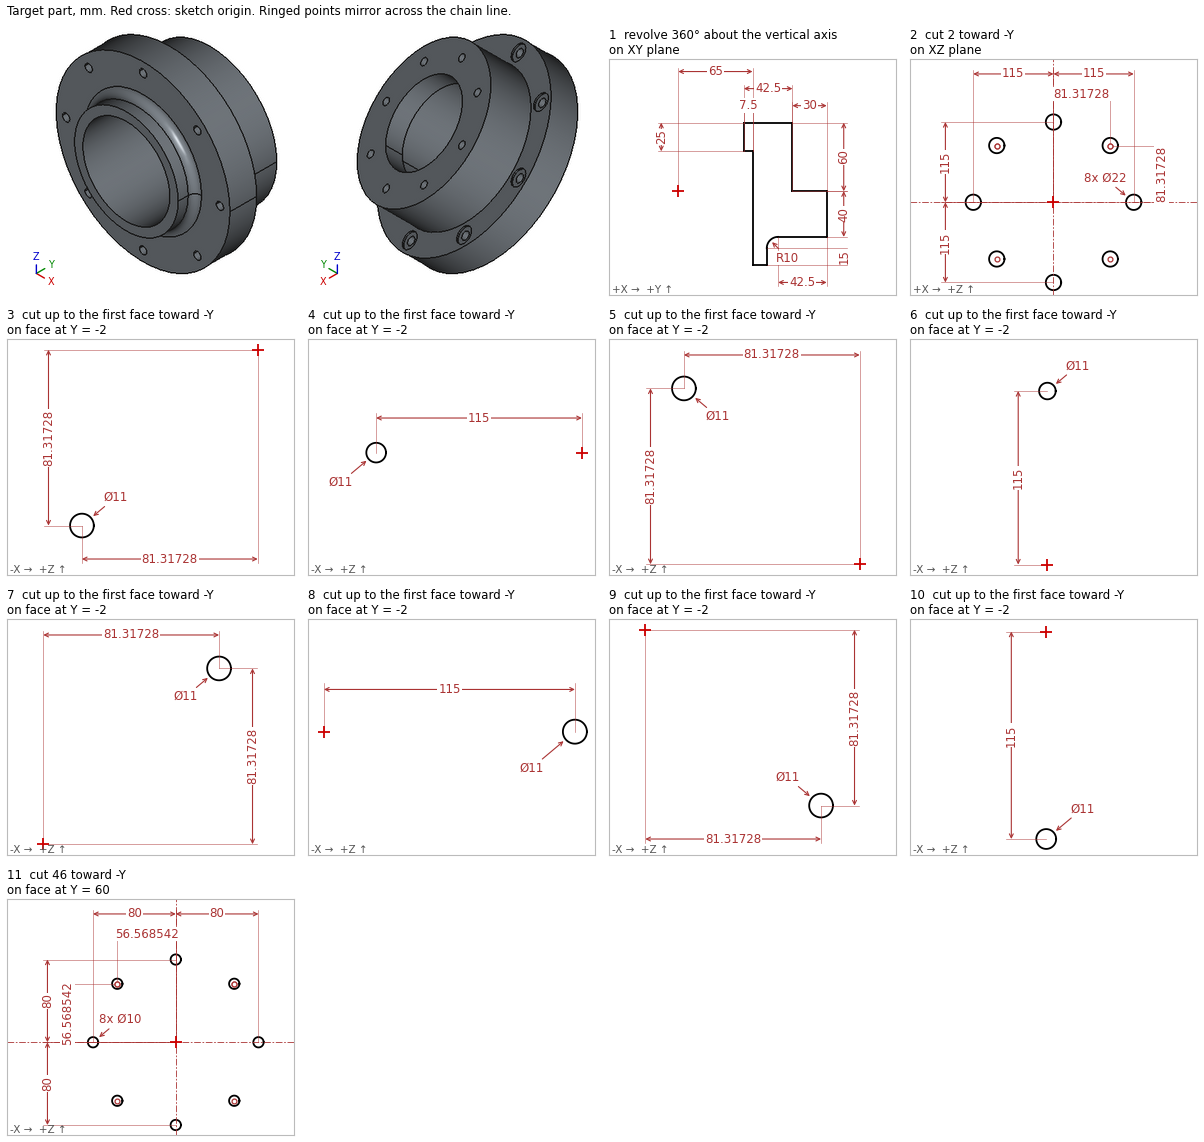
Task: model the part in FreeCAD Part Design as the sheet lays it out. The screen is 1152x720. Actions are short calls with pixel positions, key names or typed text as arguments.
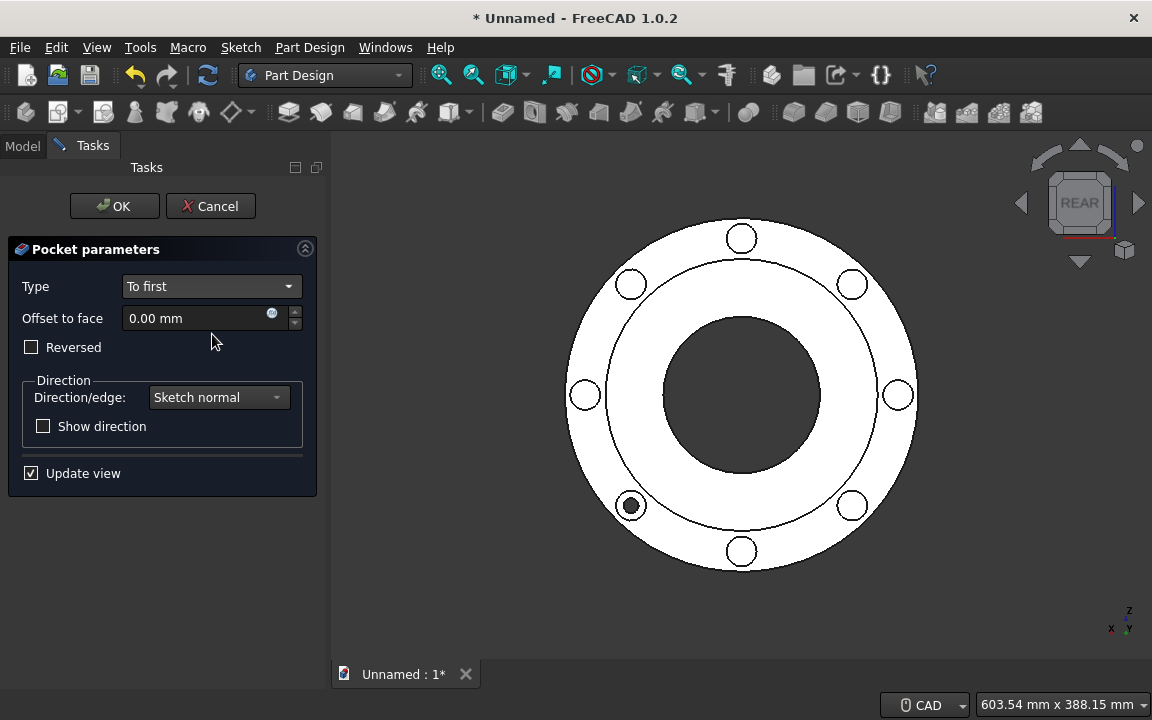
click(115, 206)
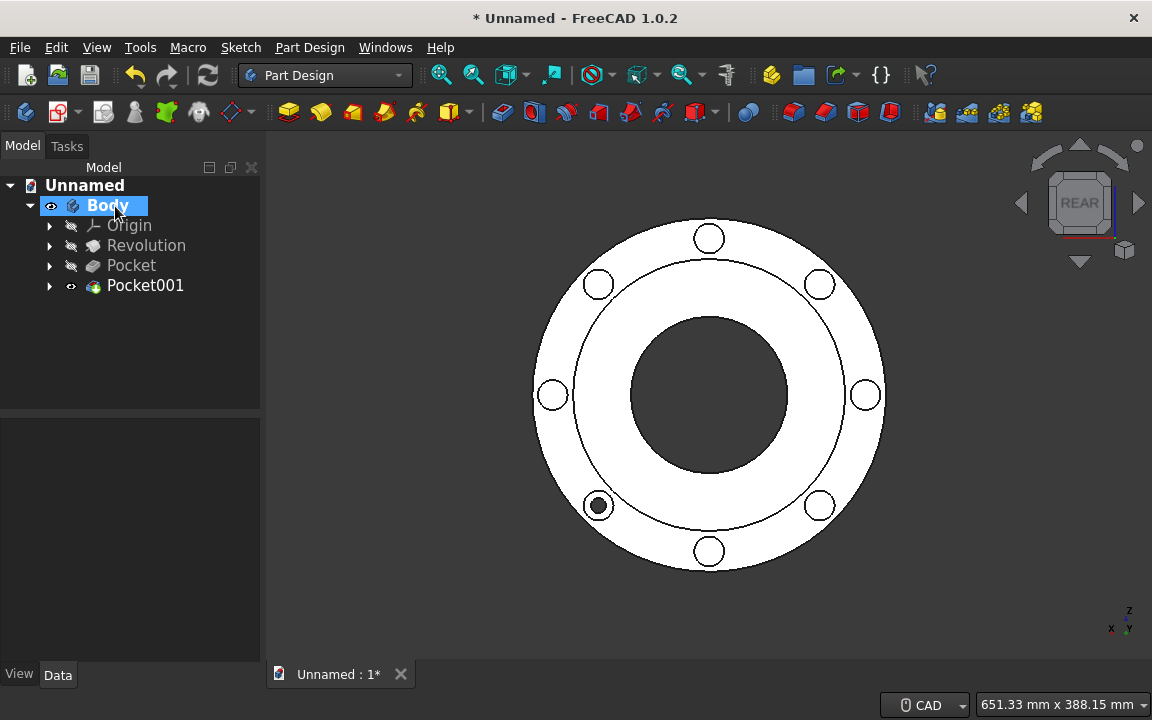
click(599, 283)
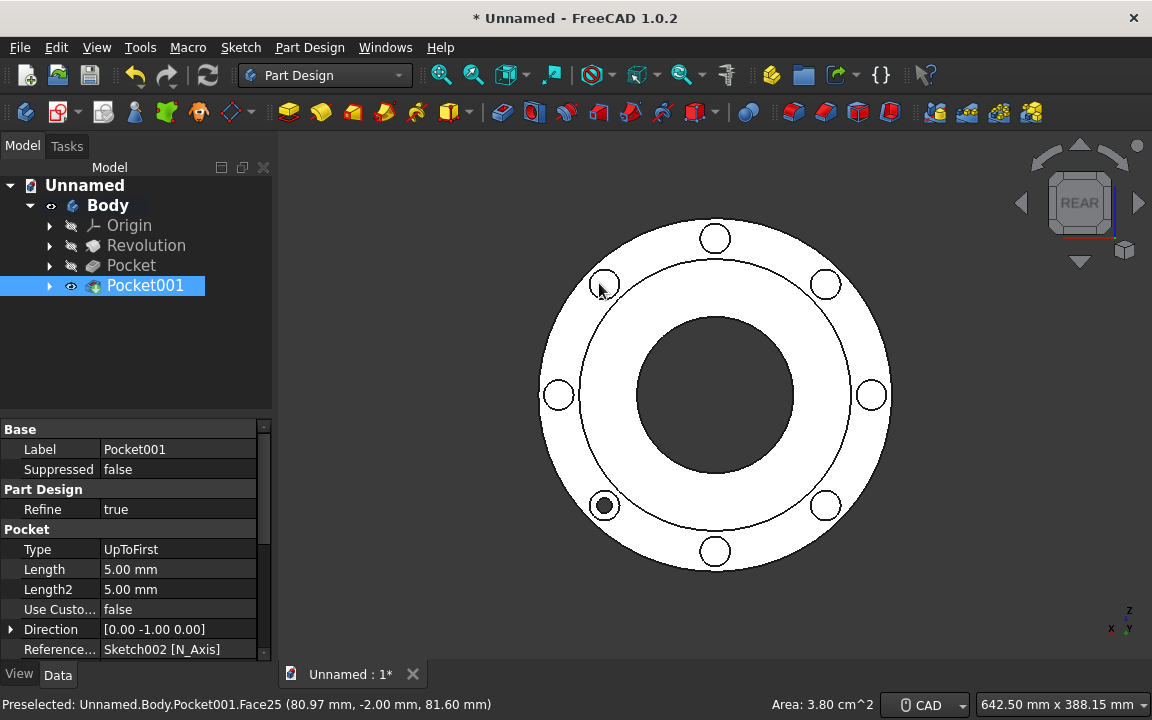
click(58, 112)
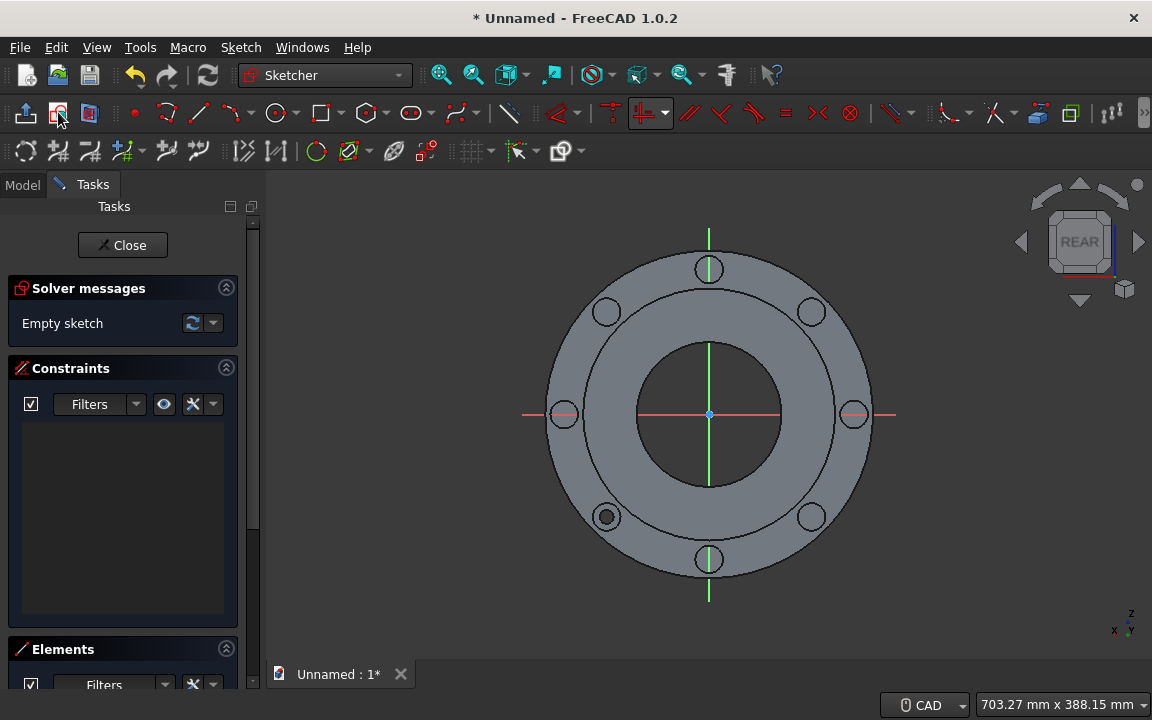
scroll(560, 415, up, 15)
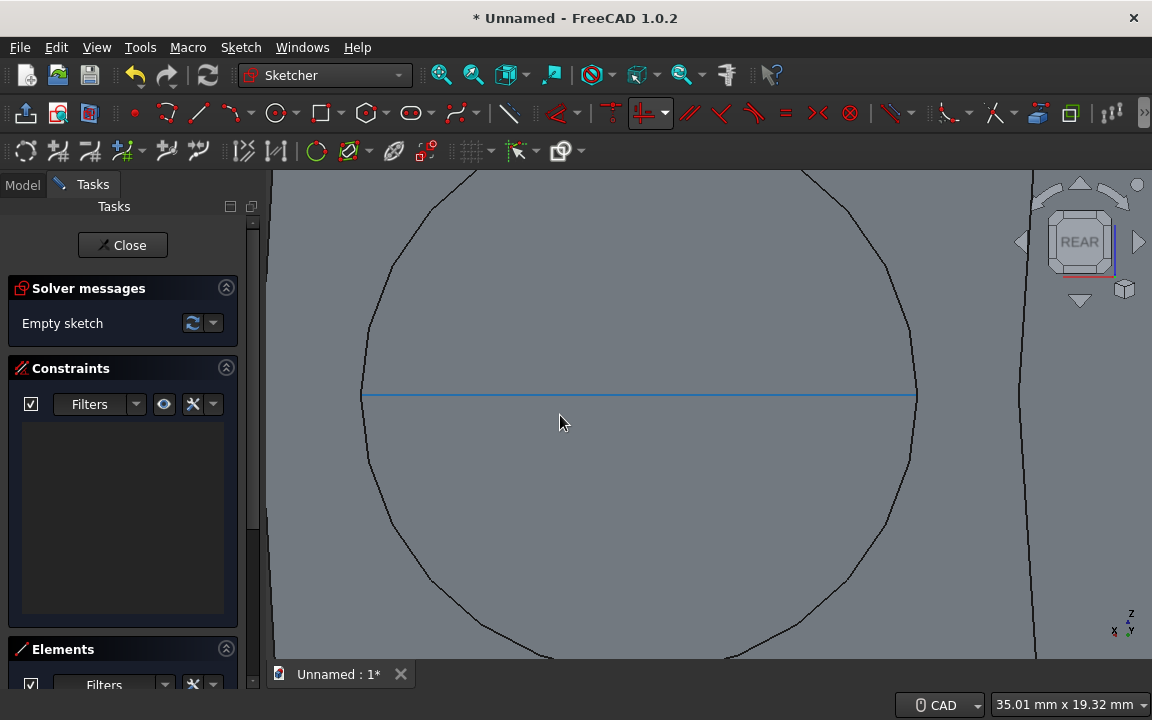
click(276, 114)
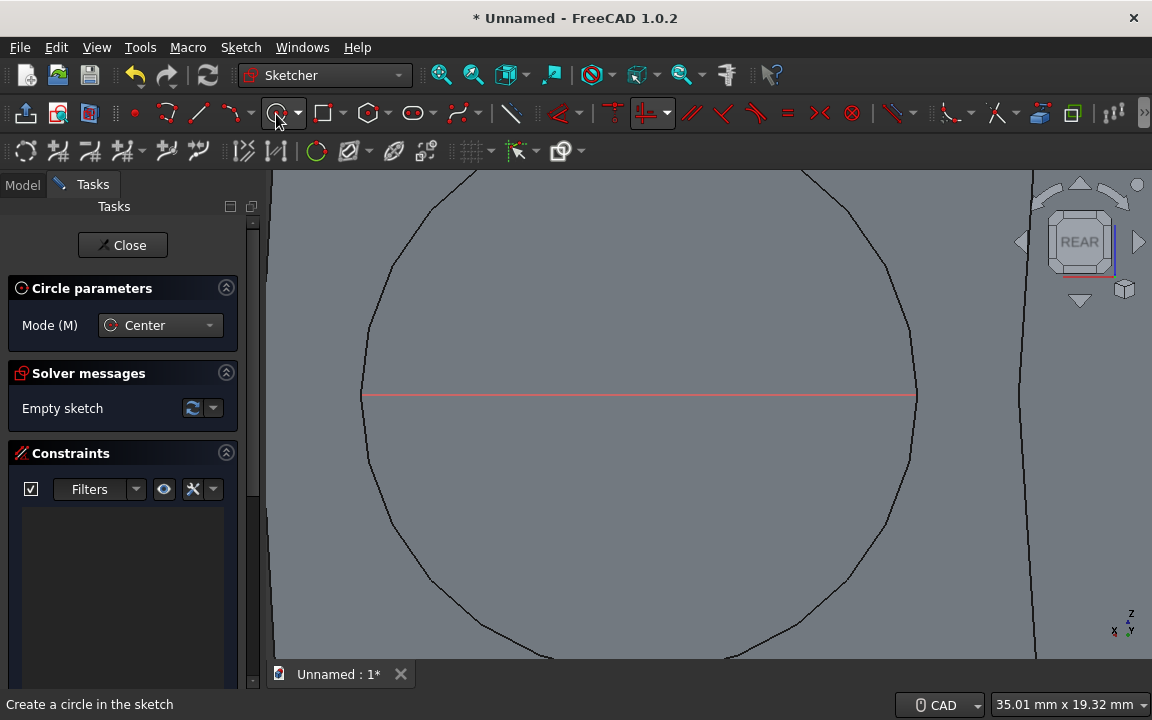
click(639, 395)
move(738, 297)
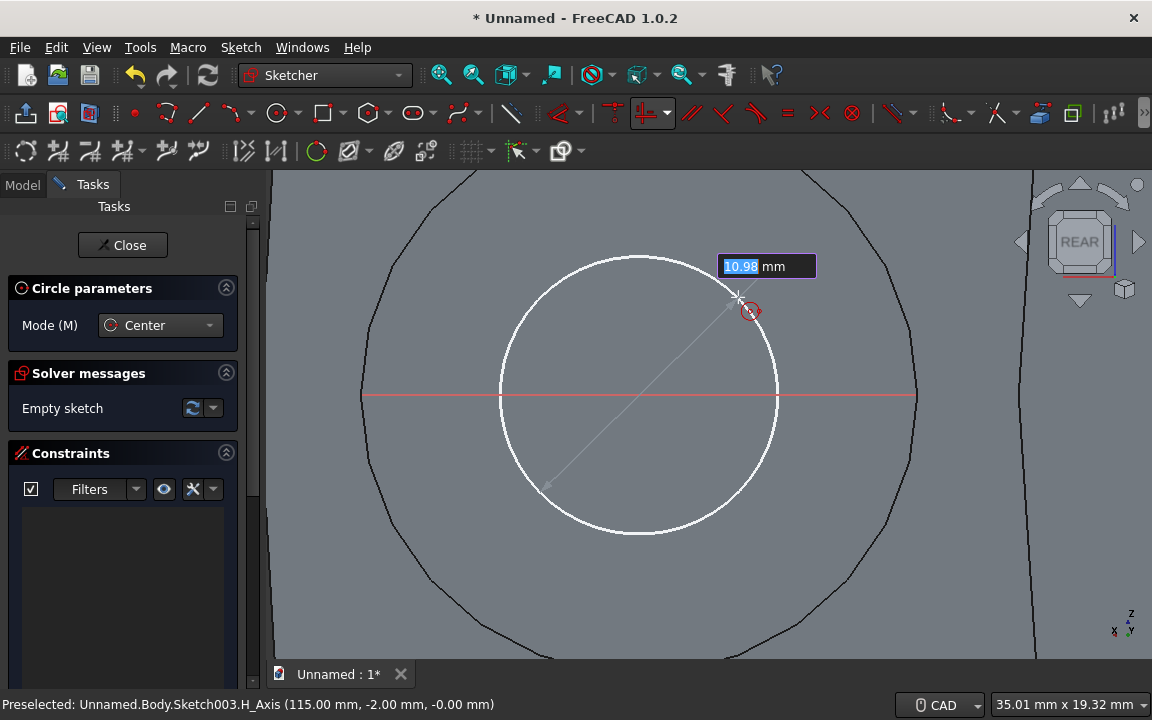
text(11)
key(Return)
key(Escape)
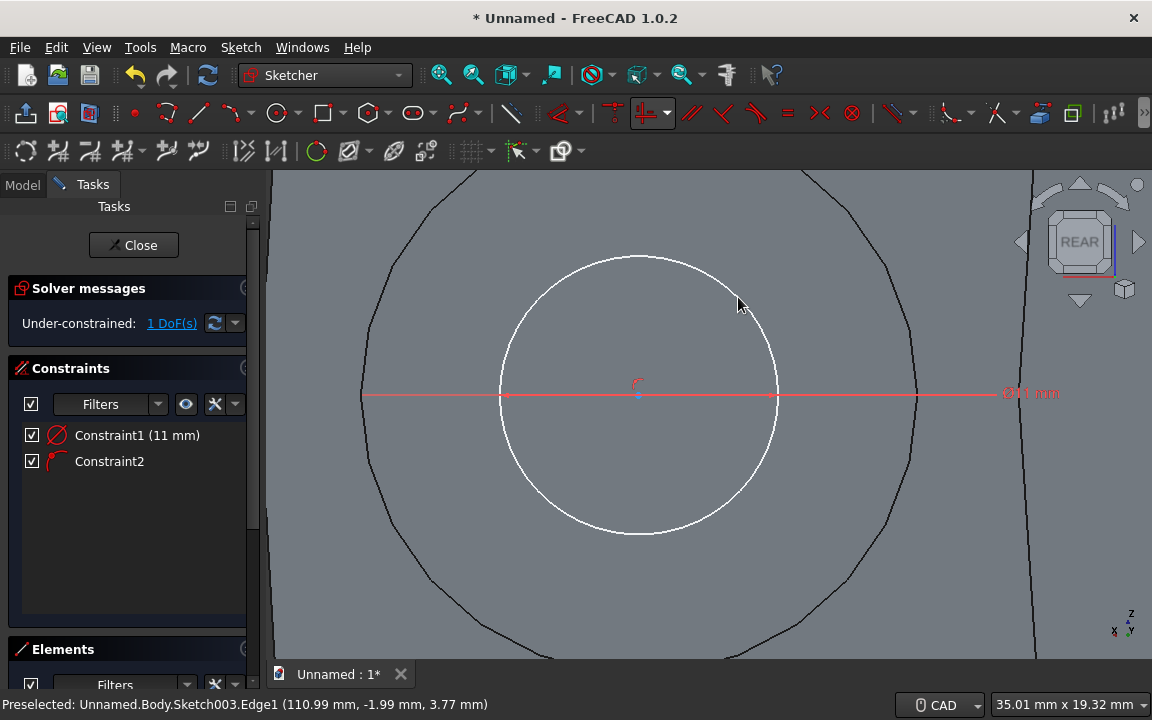
click(558, 114)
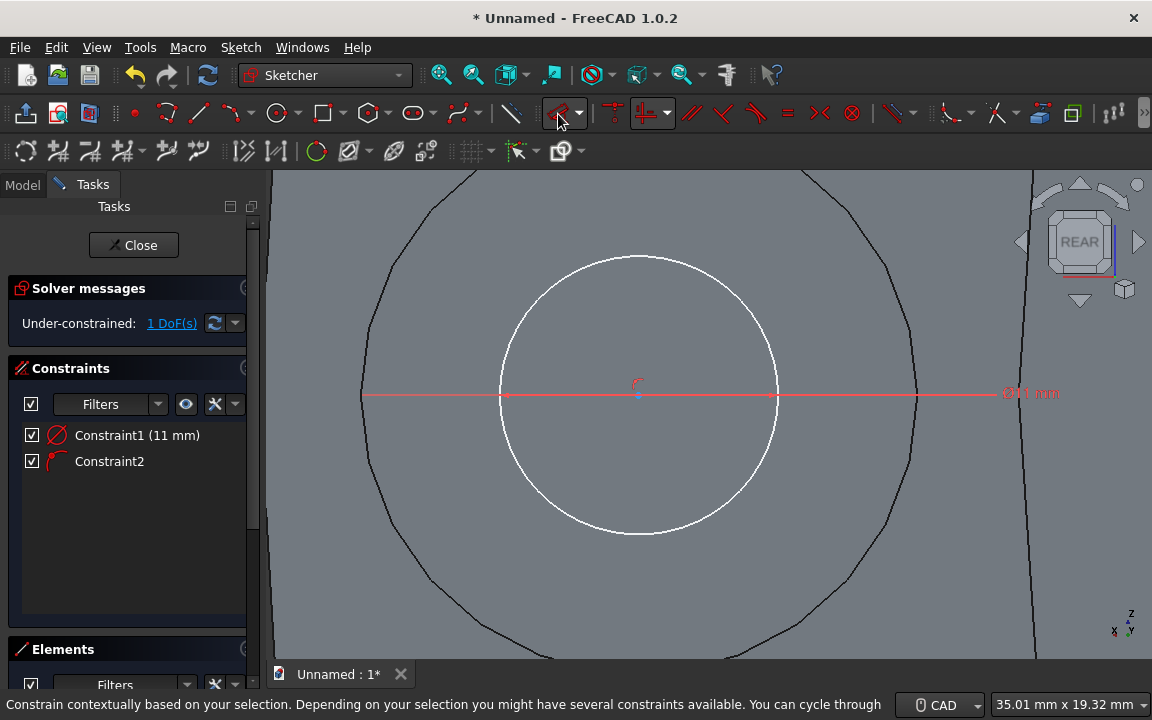
click(639, 395)
click(813, 429)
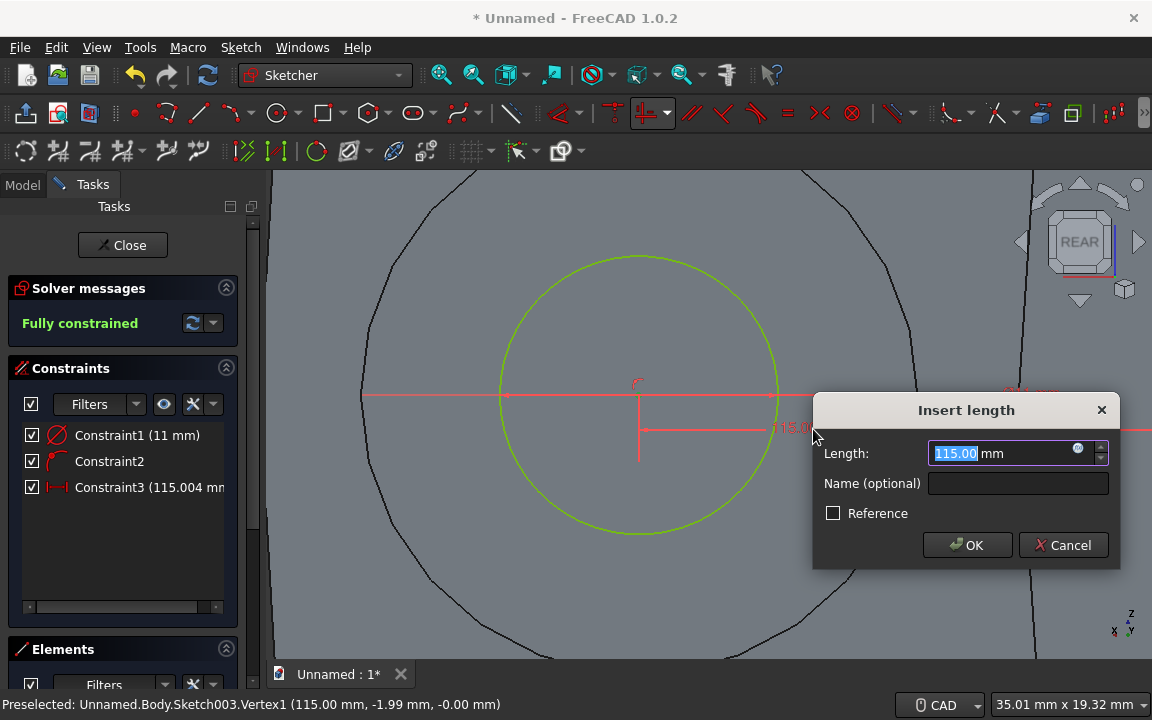
text(115)
key(Return)
key(Escape)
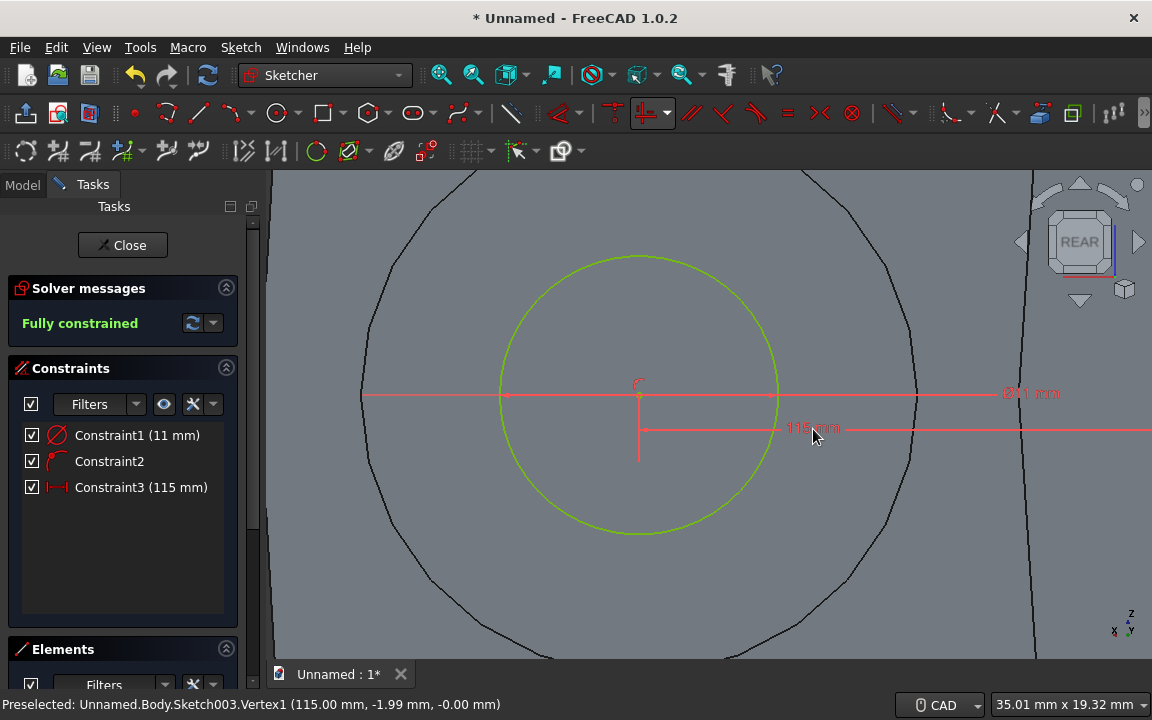
click(123, 245)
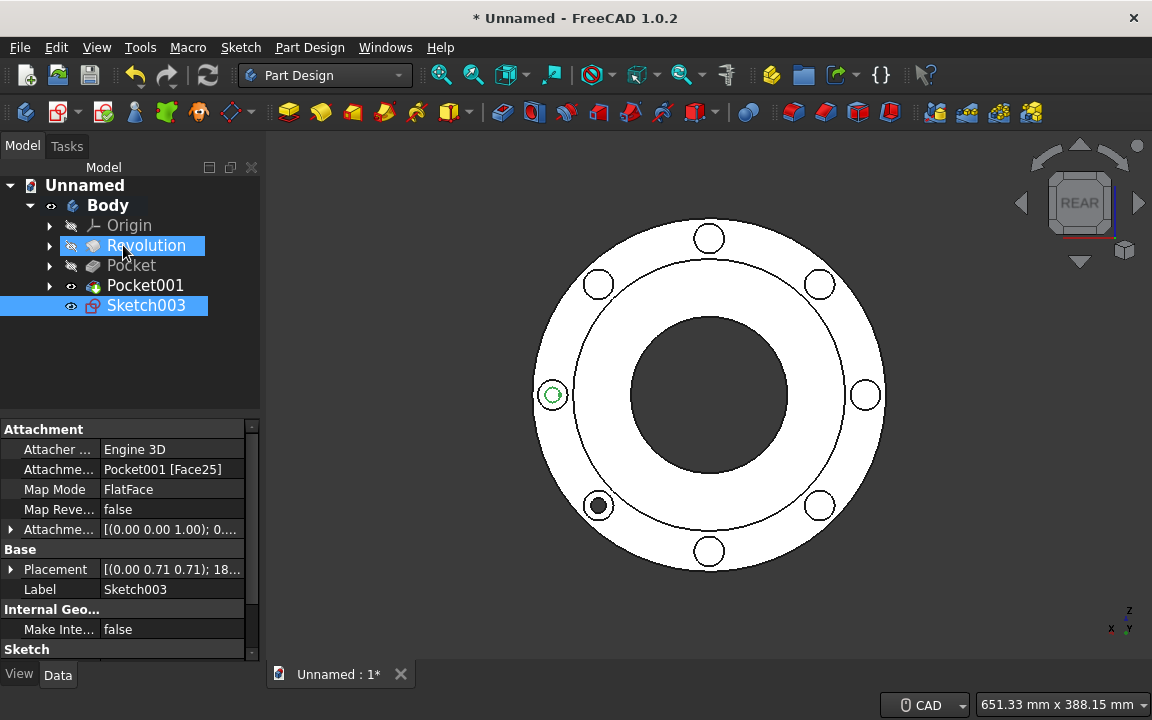
click(504, 112)